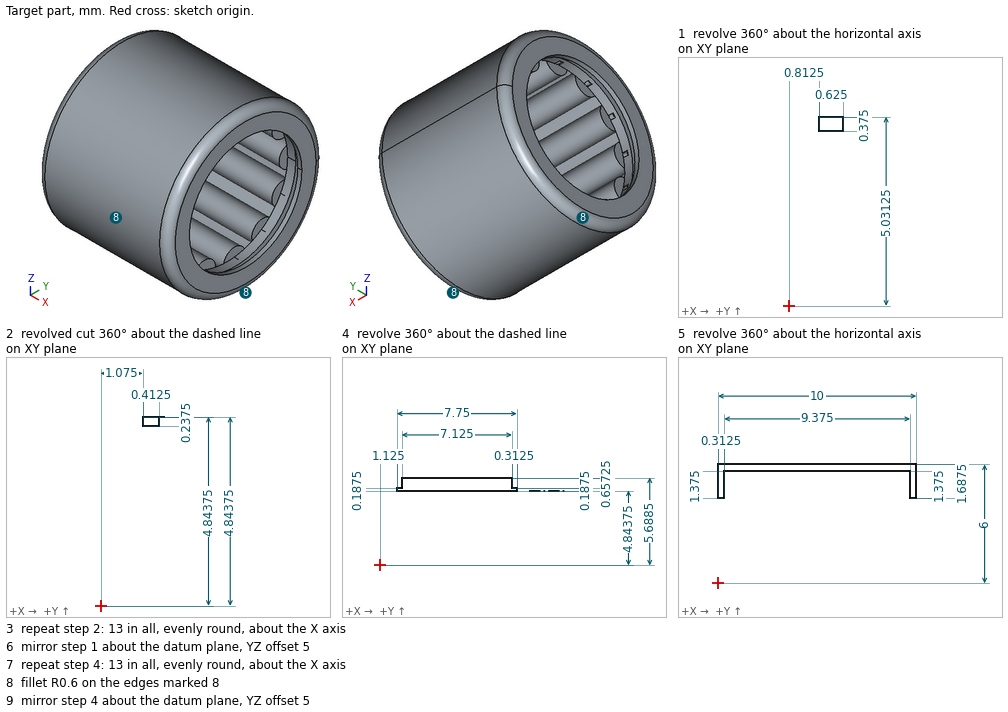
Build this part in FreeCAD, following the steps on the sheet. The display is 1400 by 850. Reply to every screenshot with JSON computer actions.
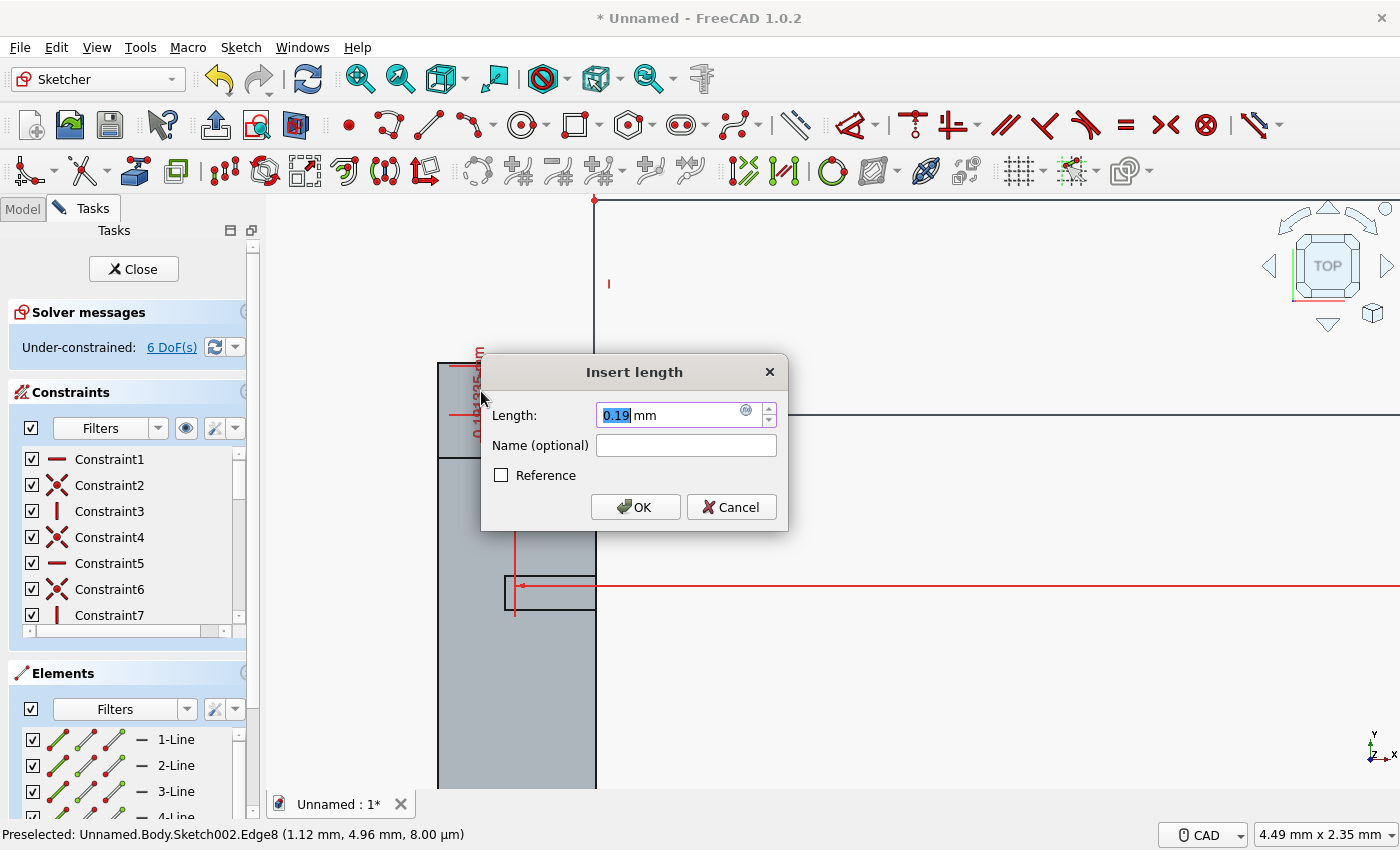
{"action": "type", "text": "0.1875"}
{"action": "key", "text": "Return"}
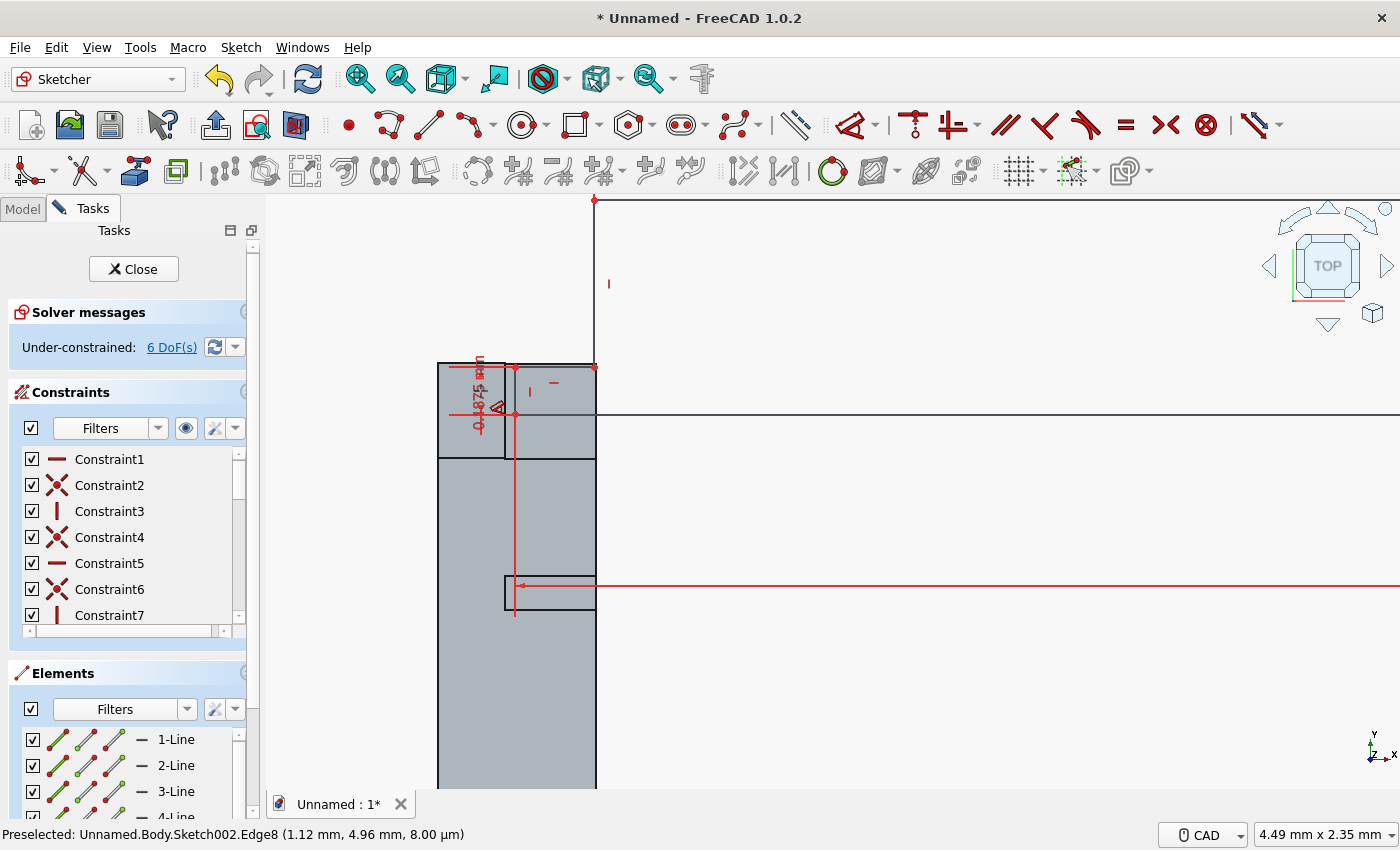
{"action": "scroll", "coordinate": [516, 384], "scroll_direction": "down", "scroll_amount": 8}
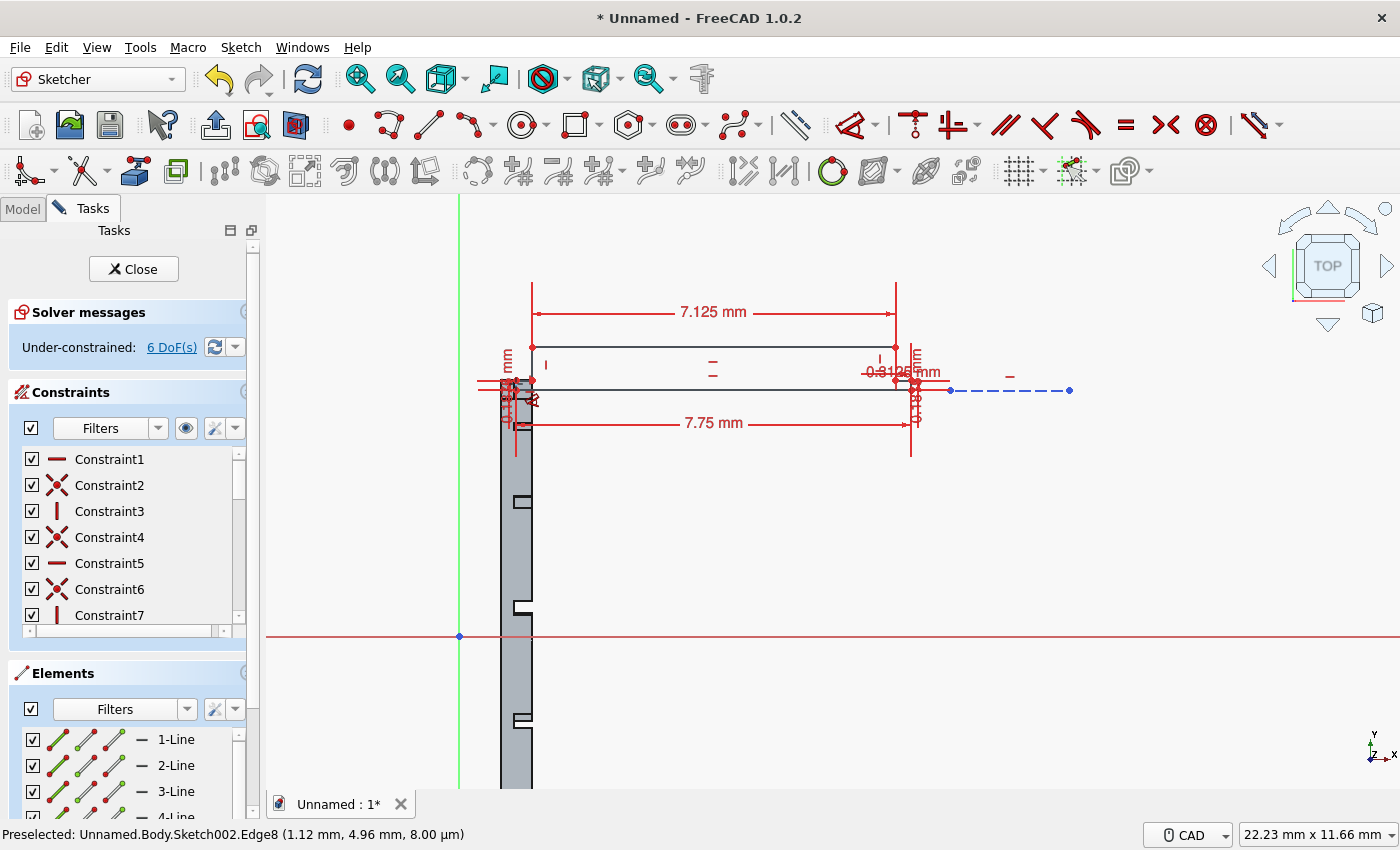
{"action": "scroll", "coordinate": [516, 390], "scroll_direction": "up", "scroll_amount": 2}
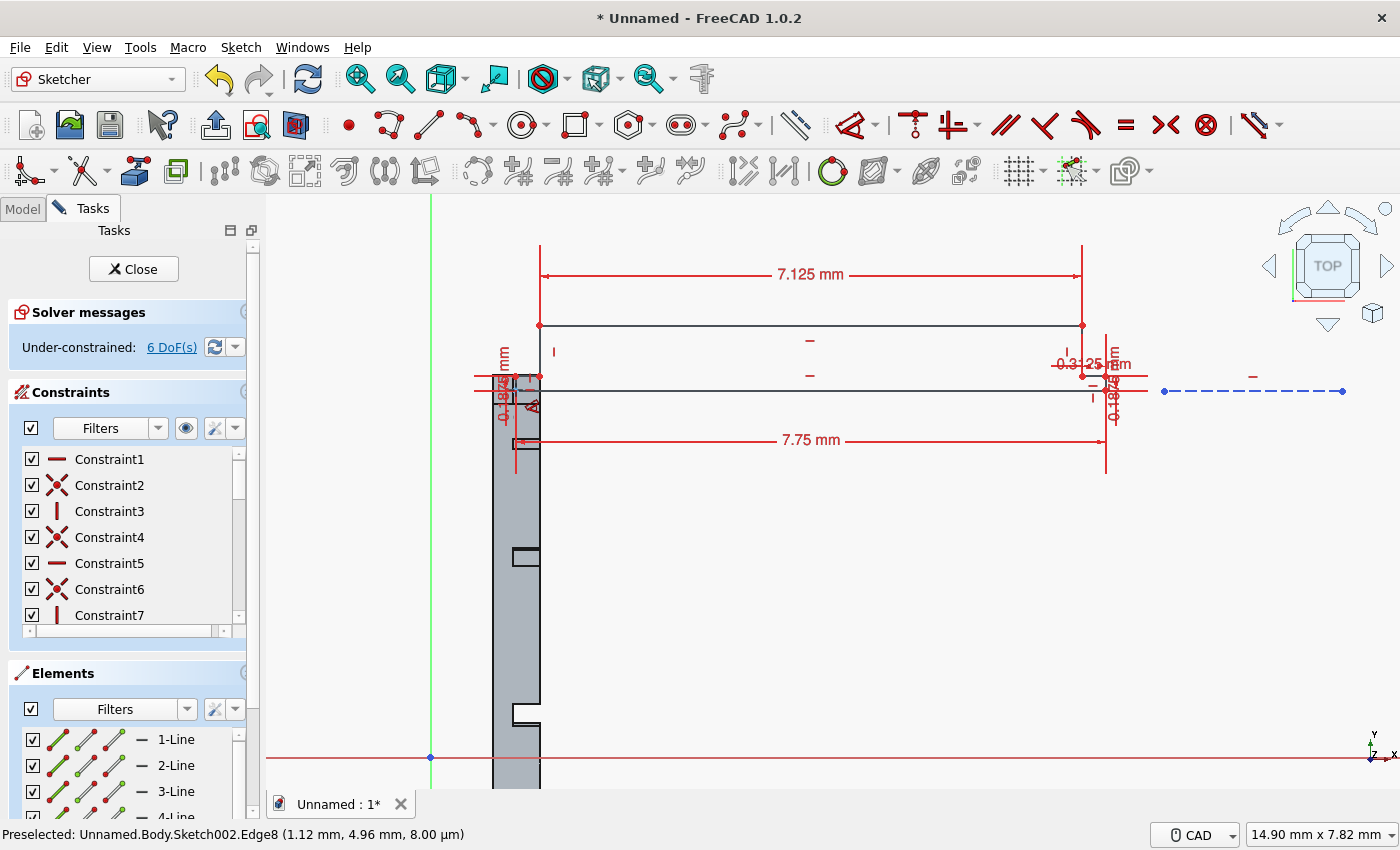
{"action": "left_click", "coordinate": [516, 391]}
{"action": "left_click", "coordinate": [473, 357]}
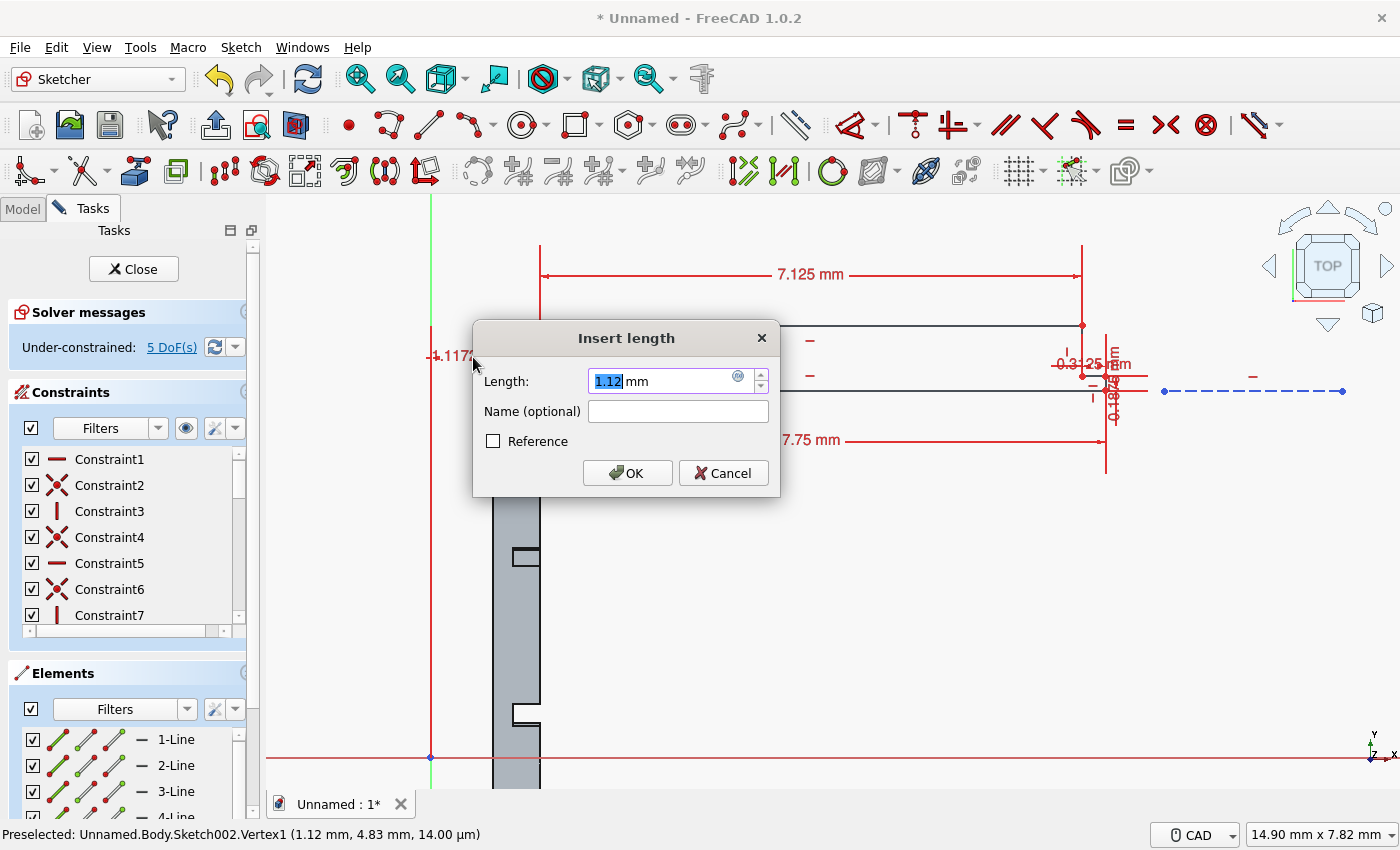
{"action": "type", "text": "1.125"}
{"action": "key", "text": "Return"}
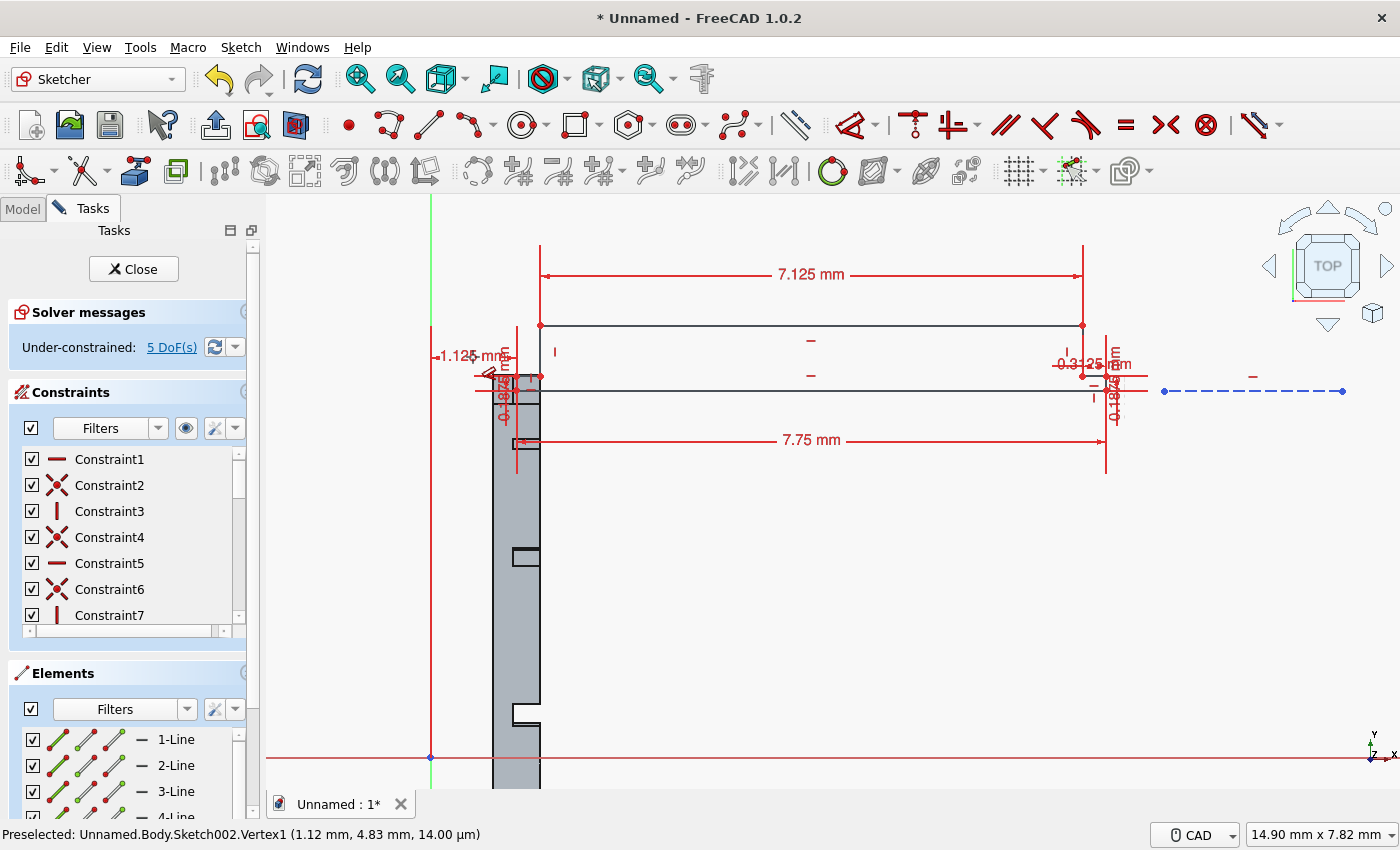
{"action": "left_click", "coordinate": [1083, 361]}
{"action": "left_click", "coordinate": [1117, 339]}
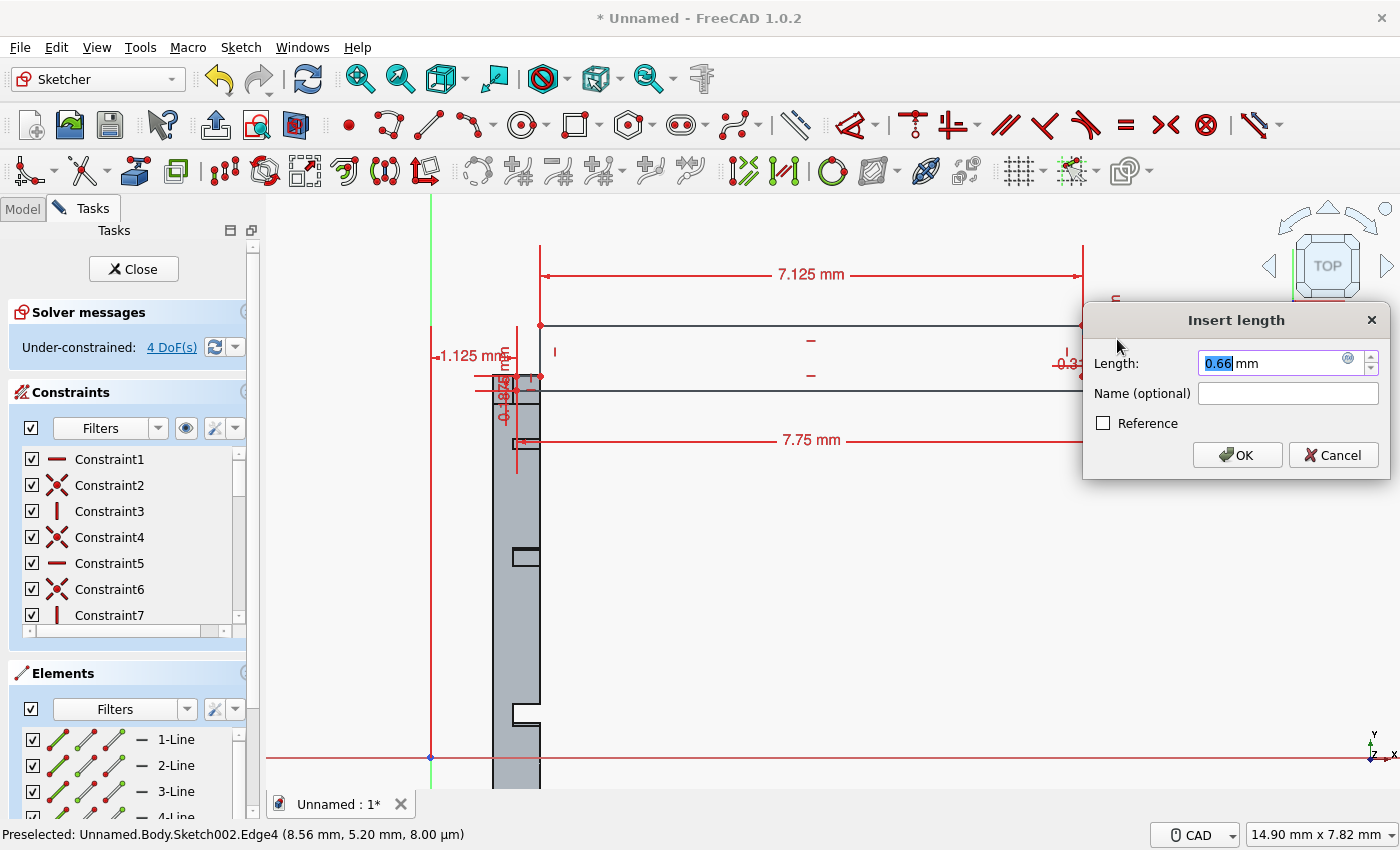
{"action": "type", "text": "0.65725"}
{"action": "key", "text": "Return"}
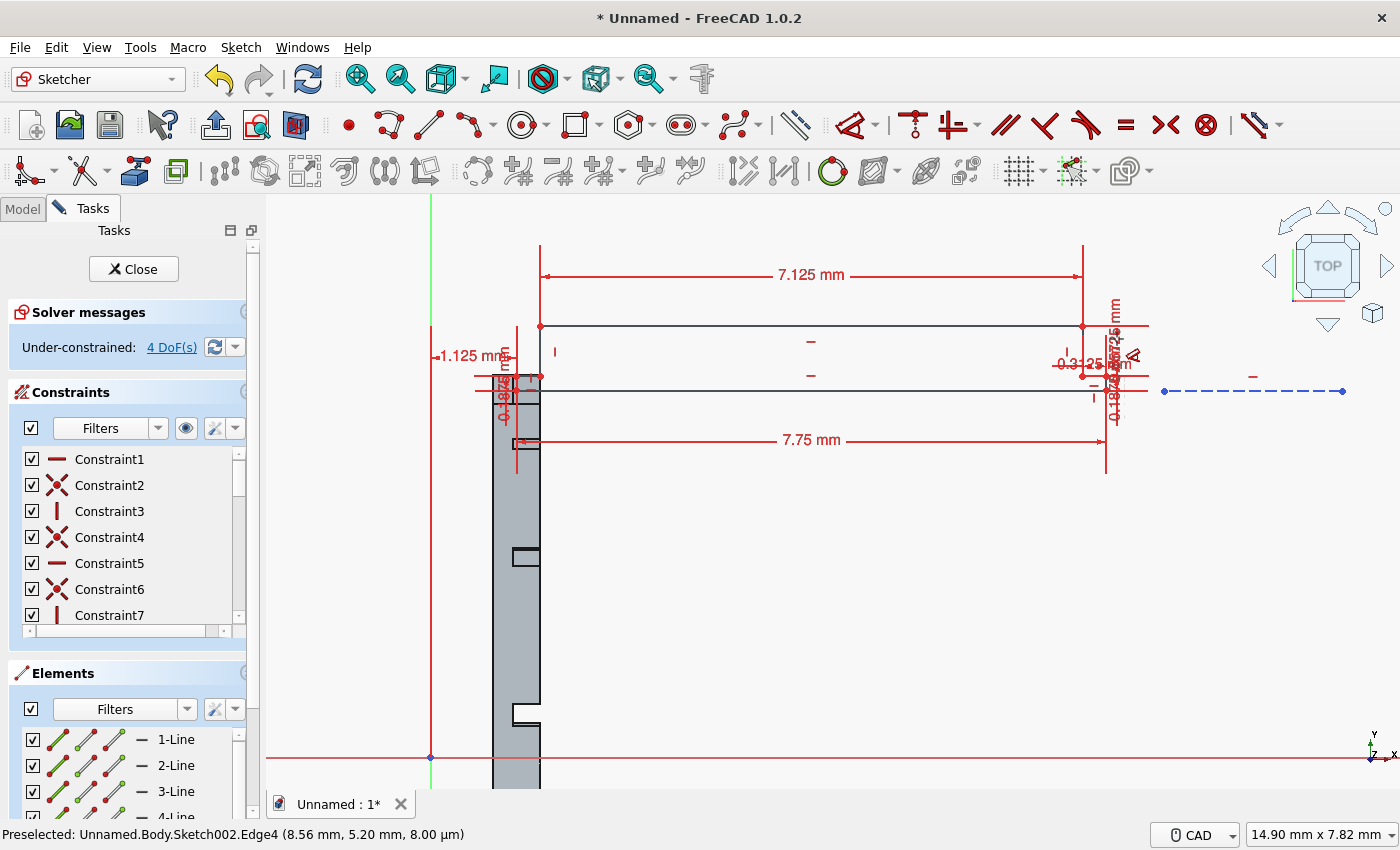
{"action": "left_click", "coordinate": [1083, 326]}
{"action": "left_click", "coordinate": [397, 542]}